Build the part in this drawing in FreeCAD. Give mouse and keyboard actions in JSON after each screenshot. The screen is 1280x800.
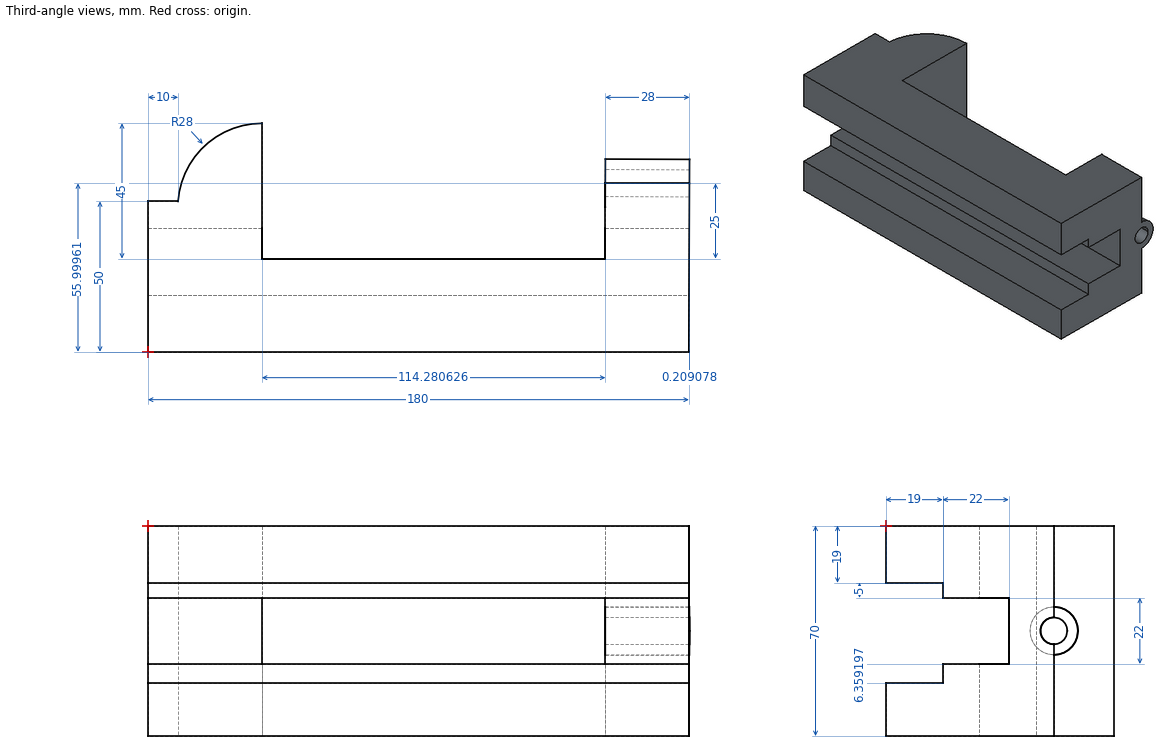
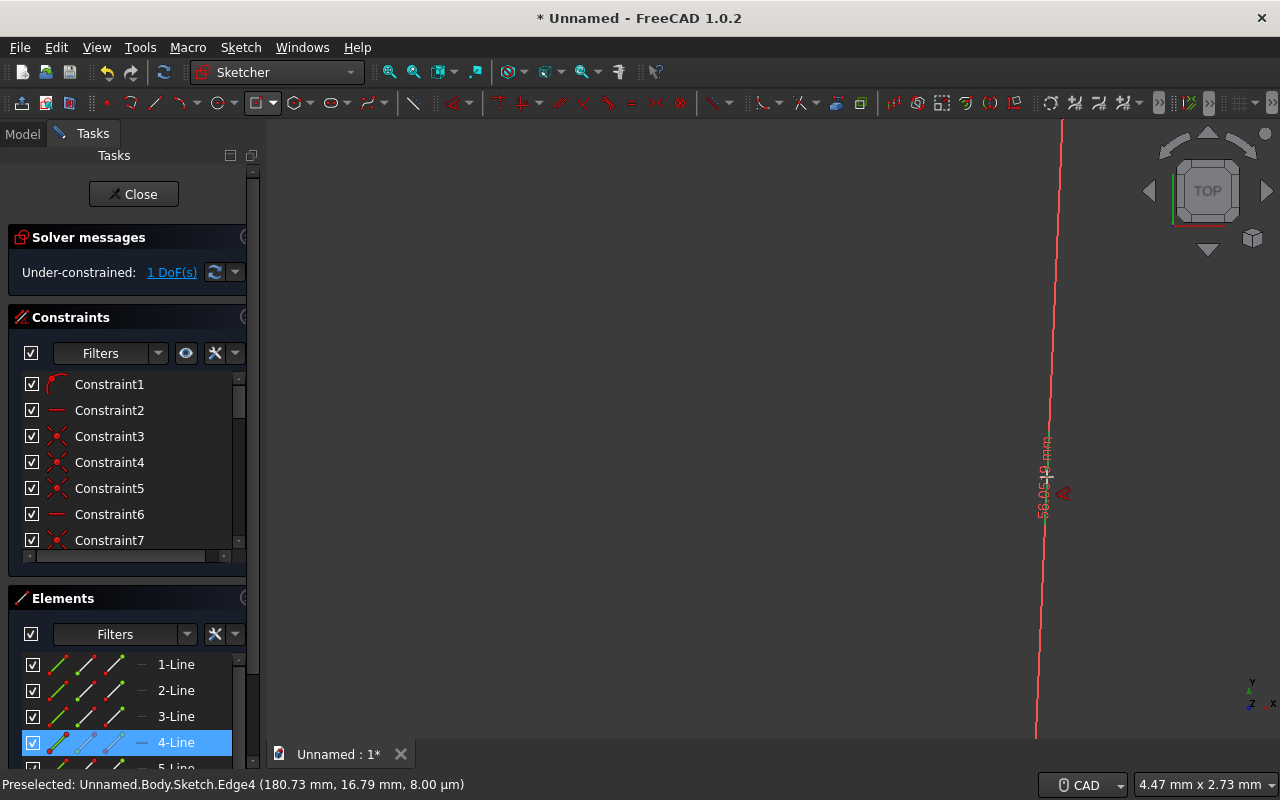
{"action": "key", "text": "Escape"}
{"action": "key", "text": "Escape"}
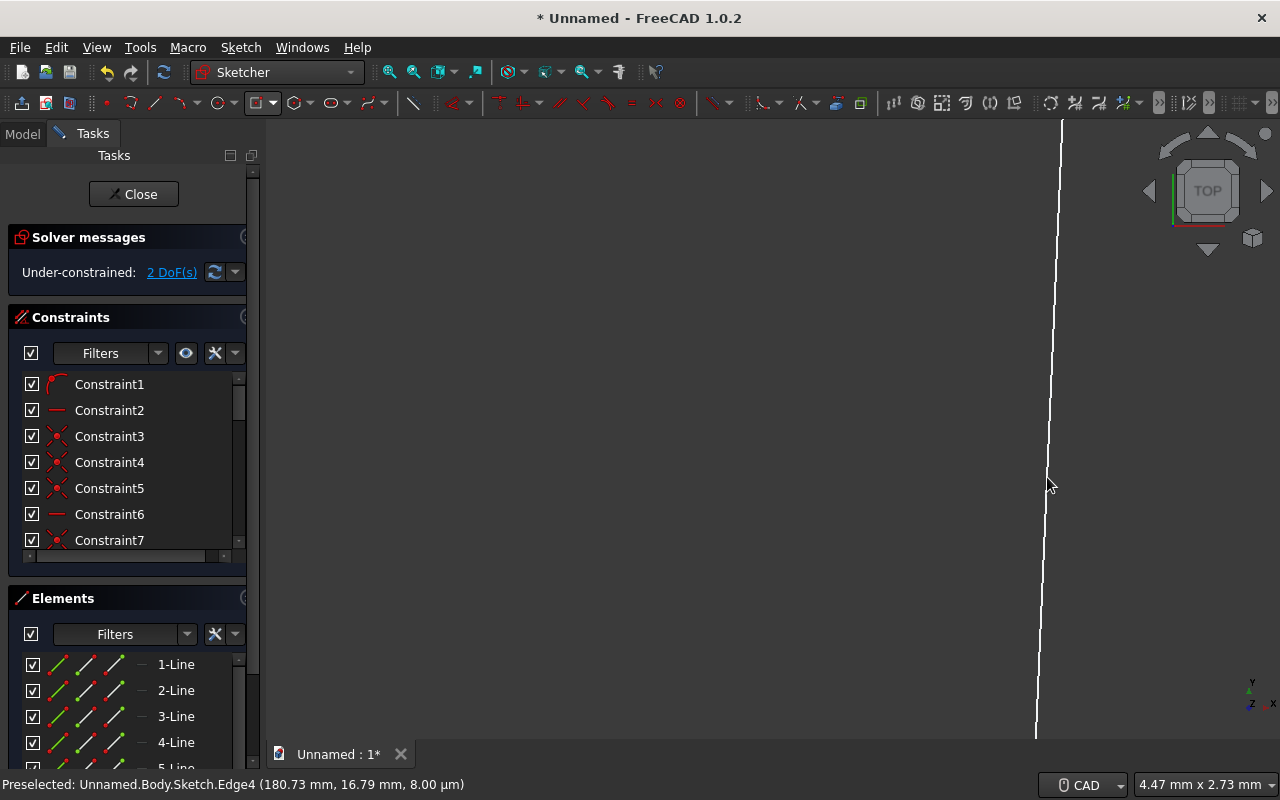
{"action": "left_click", "coordinate": [1047, 477]}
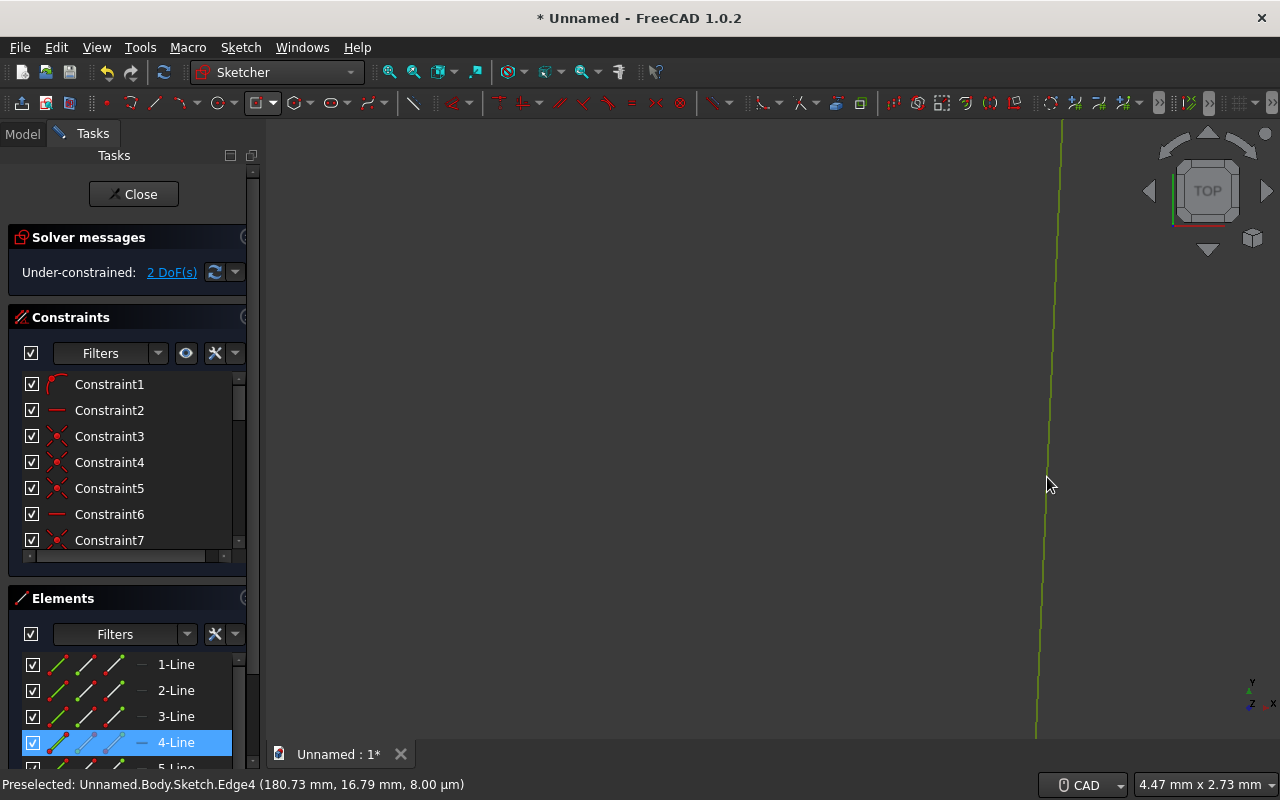
{"action": "key", "text": "l"}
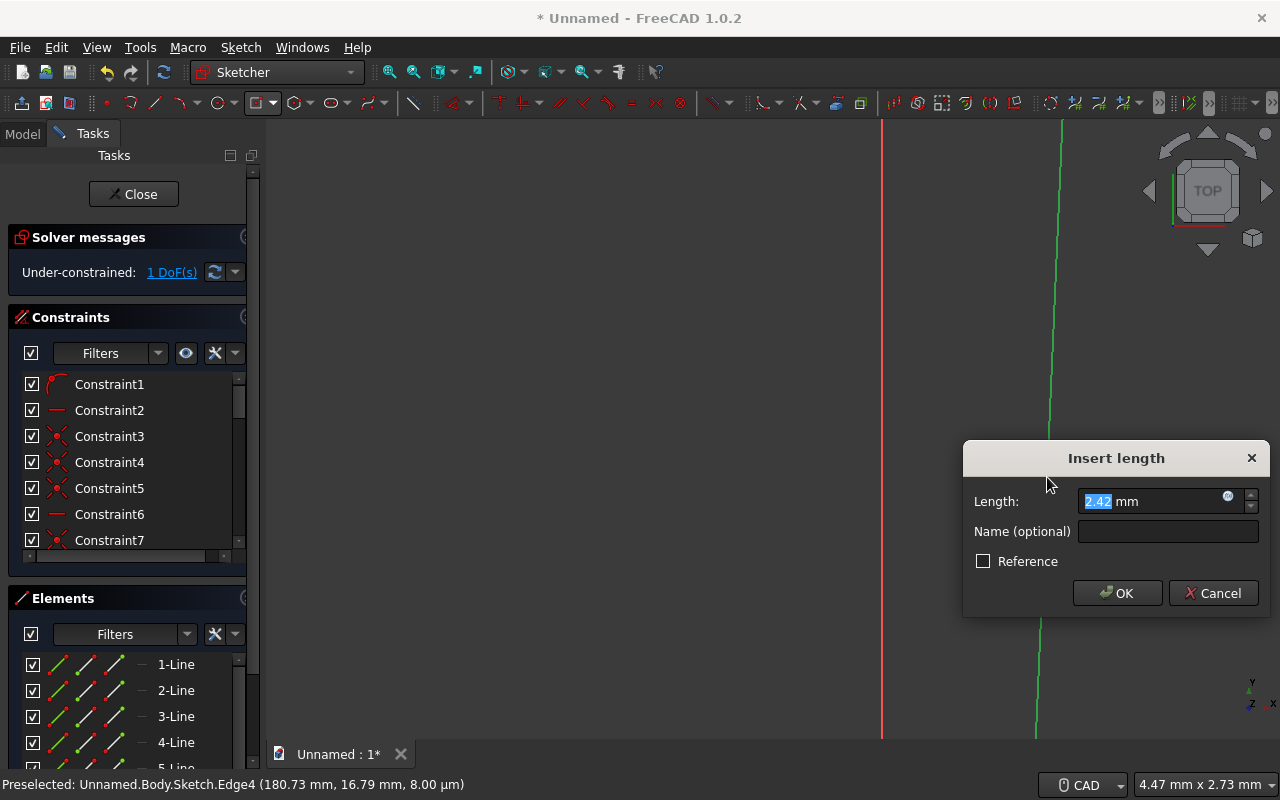
{"action": "type", "text": "0.209078"}
{"action": "key", "text": "Return"}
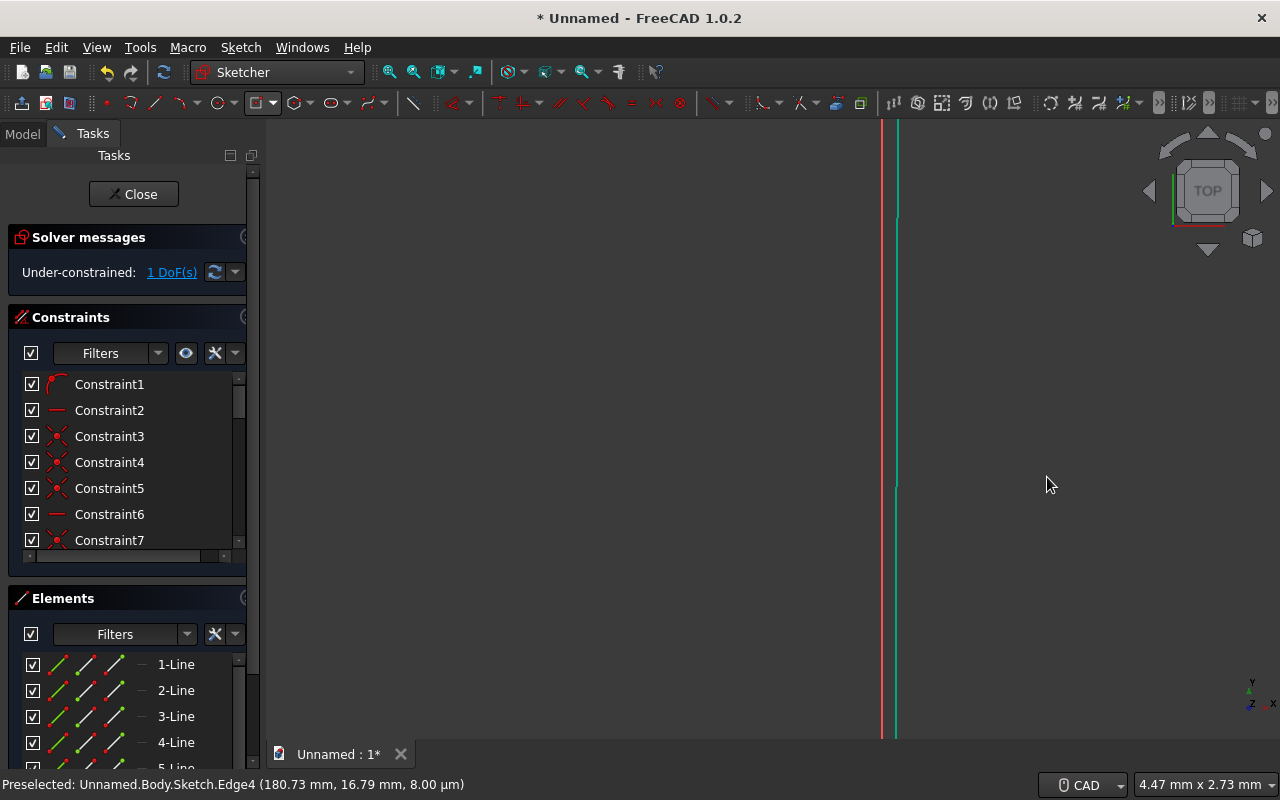
{"action": "scroll", "coordinate": [704, 429], "scroll_direction": "down", "scroll_amount": 15}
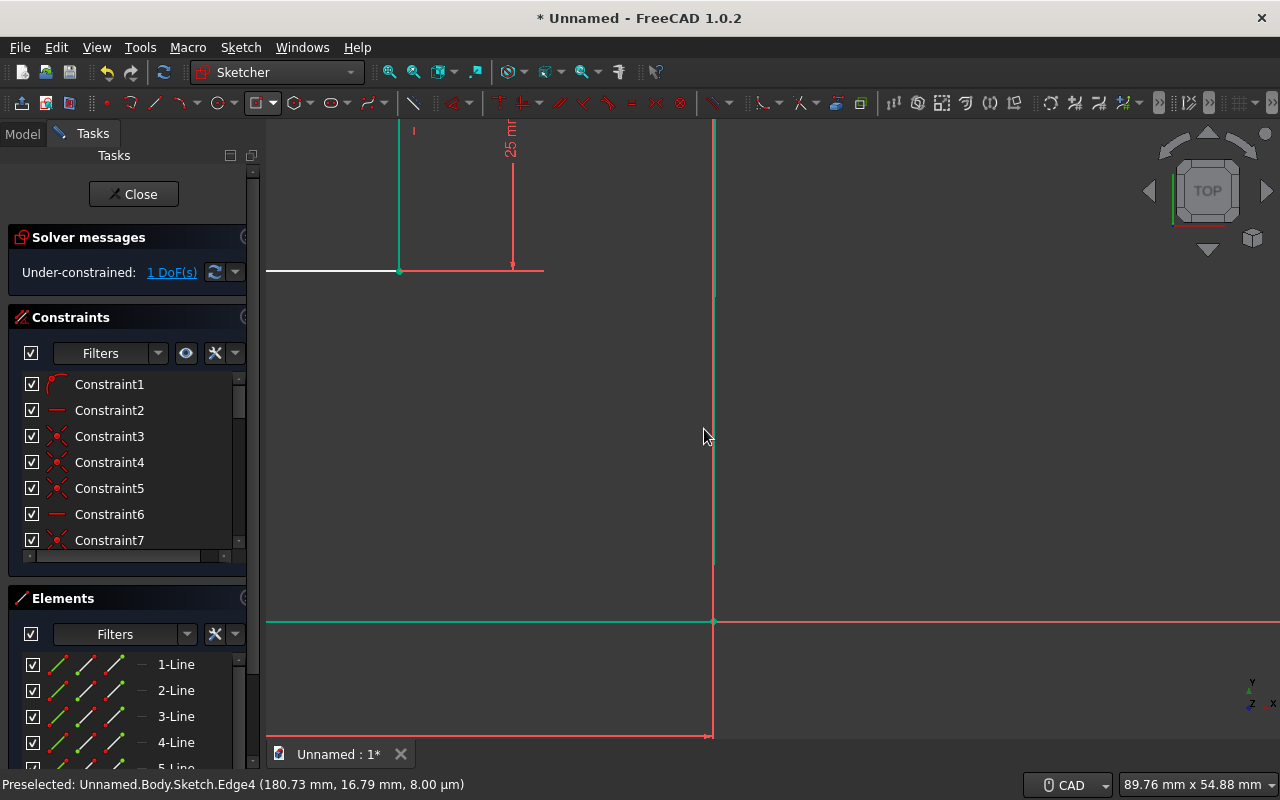
{"action": "scroll", "coordinate": [1115, 531], "scroll_direction": "down", "scroll_amount": 6}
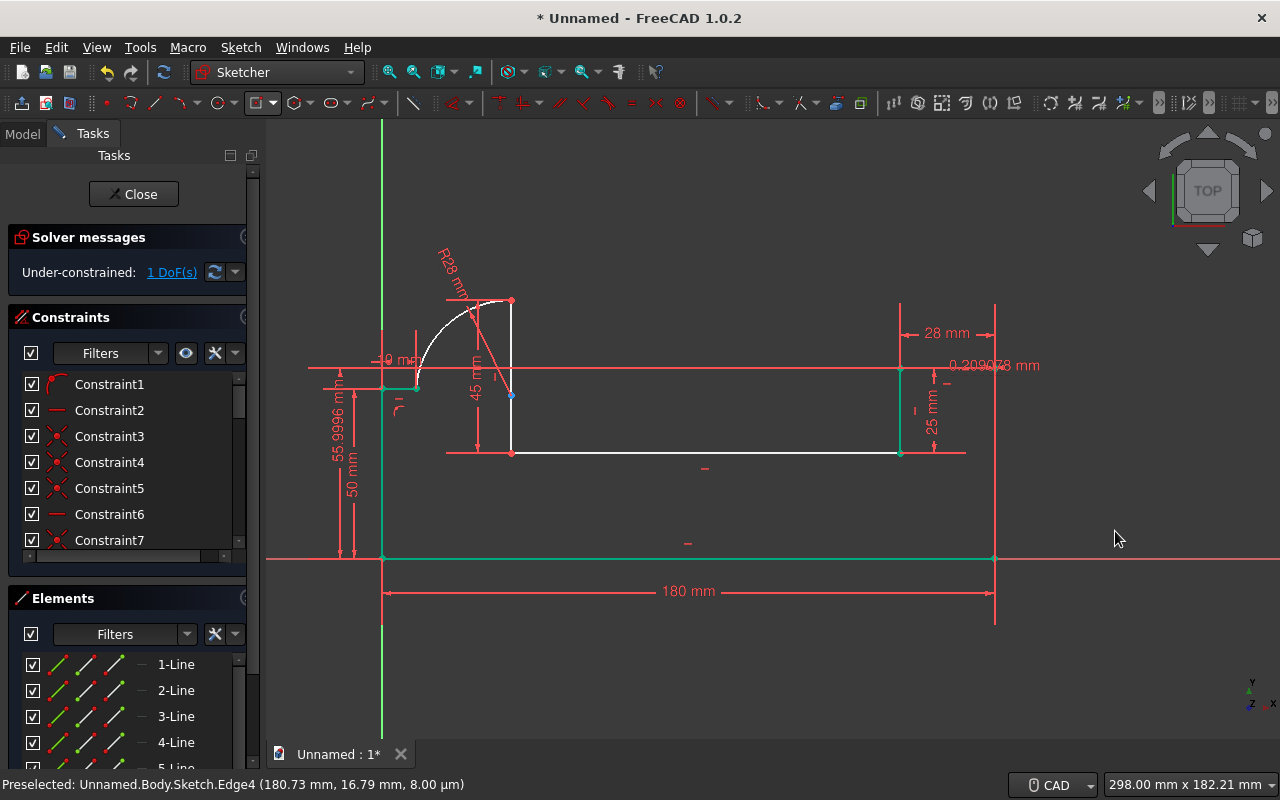
{"action": "left_click", "coordinate": [783, 453]}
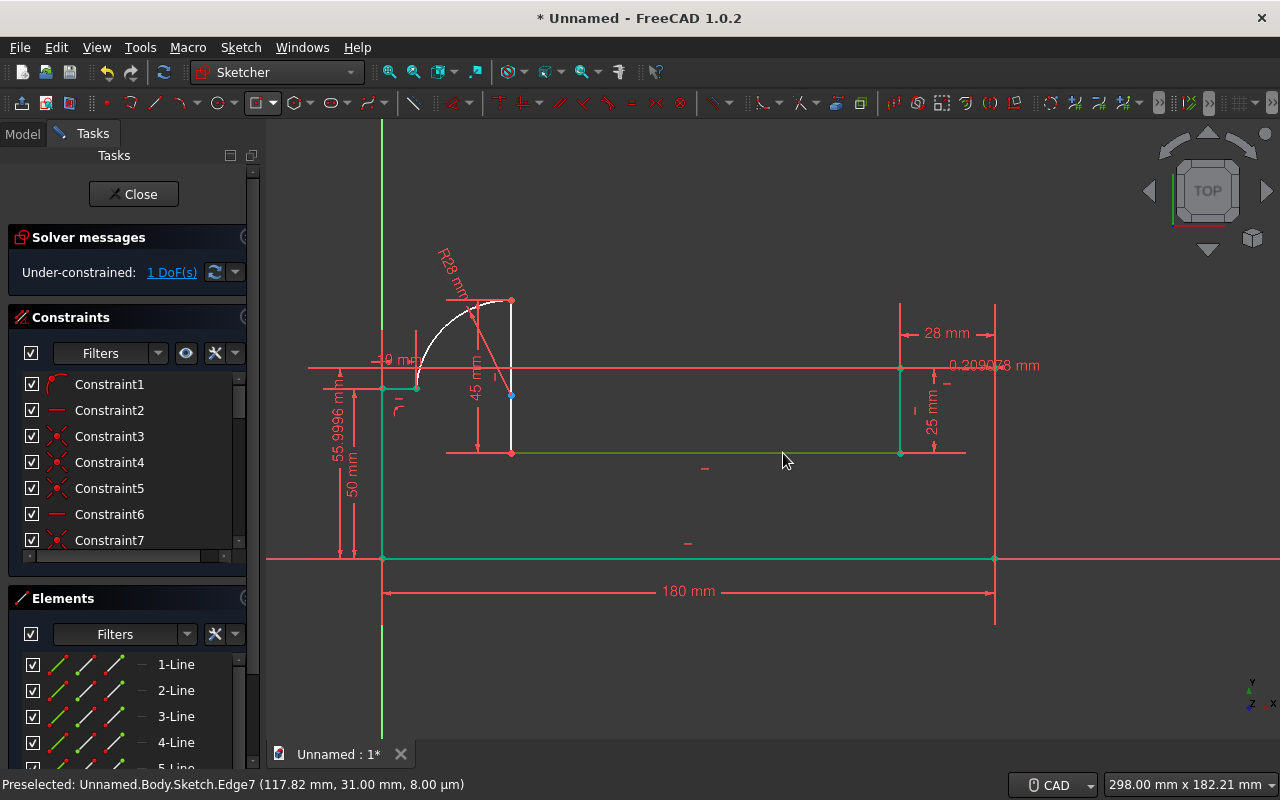
{"action": "key", "text": "l"}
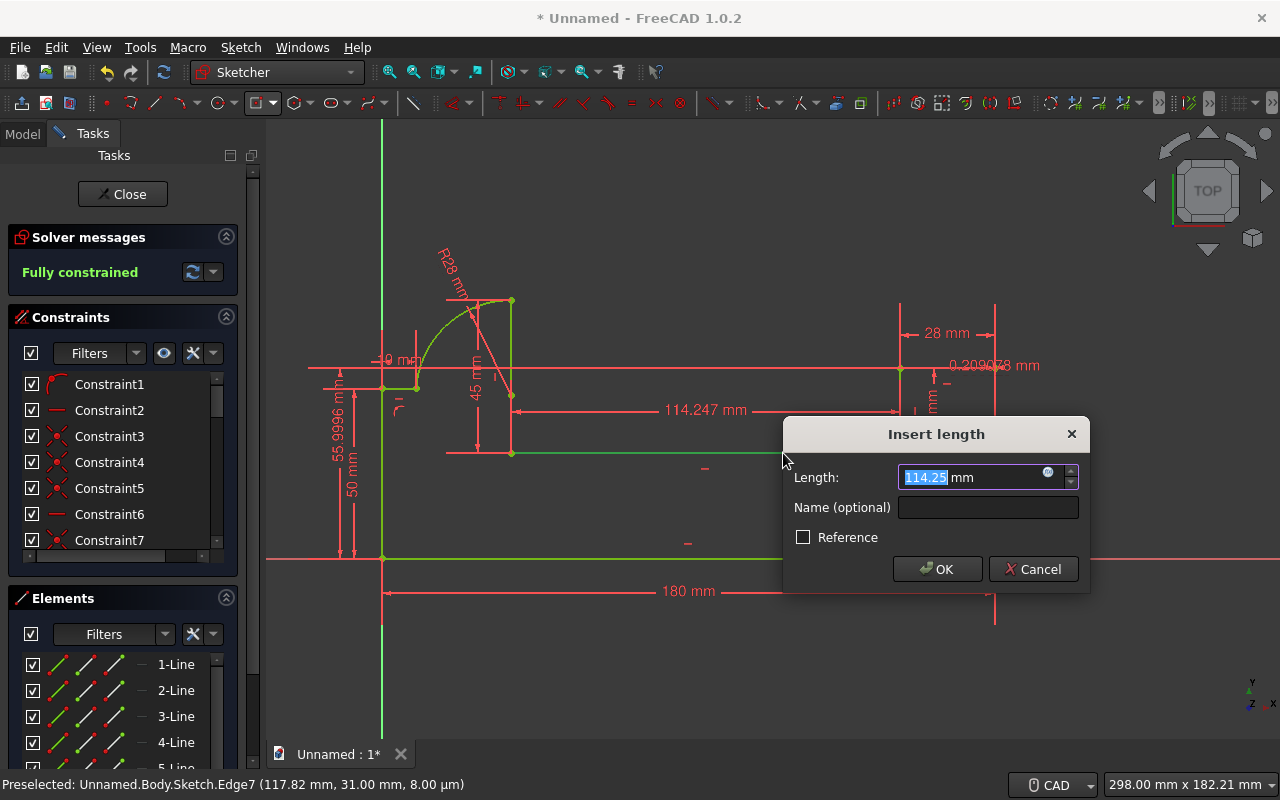
{"action": "type", "text": "114.280626"}
{"action": "key", "text": "Return"}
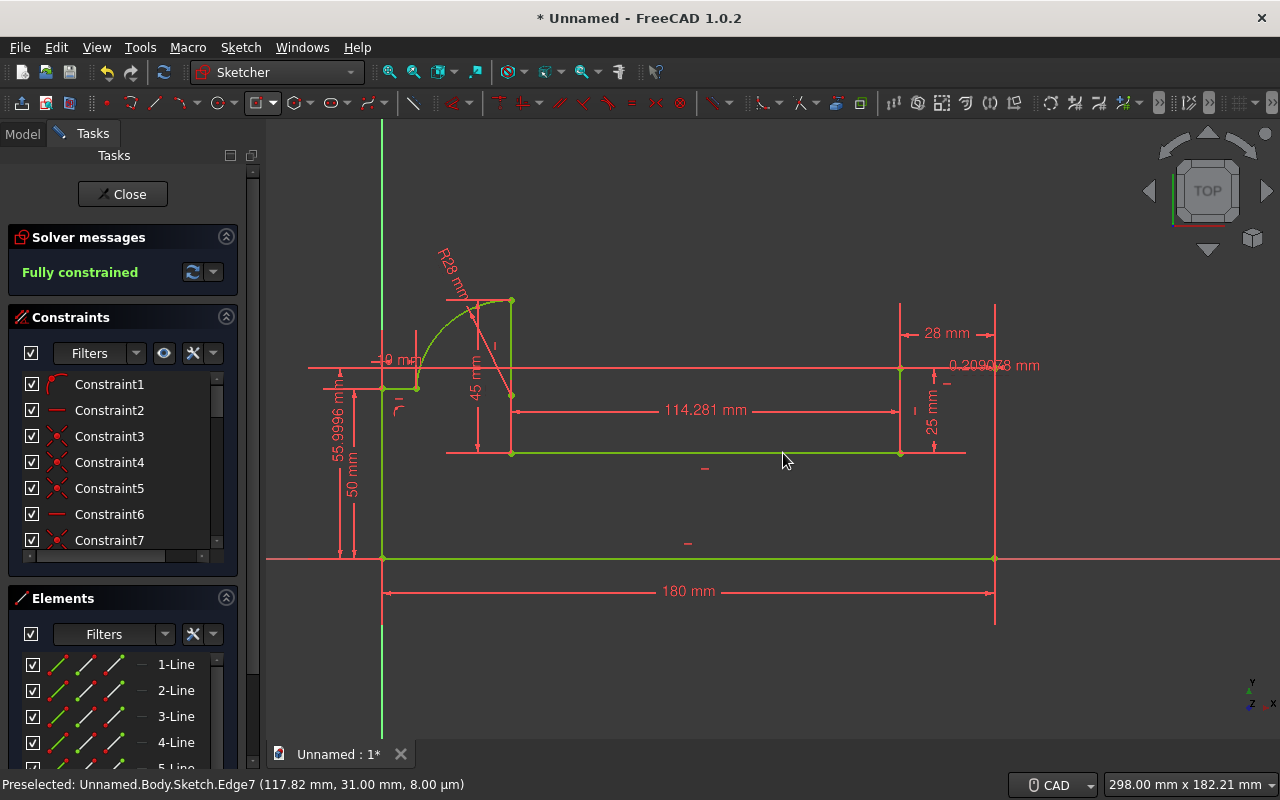
{"action": "left_click", "coordinate": [123, 194]}